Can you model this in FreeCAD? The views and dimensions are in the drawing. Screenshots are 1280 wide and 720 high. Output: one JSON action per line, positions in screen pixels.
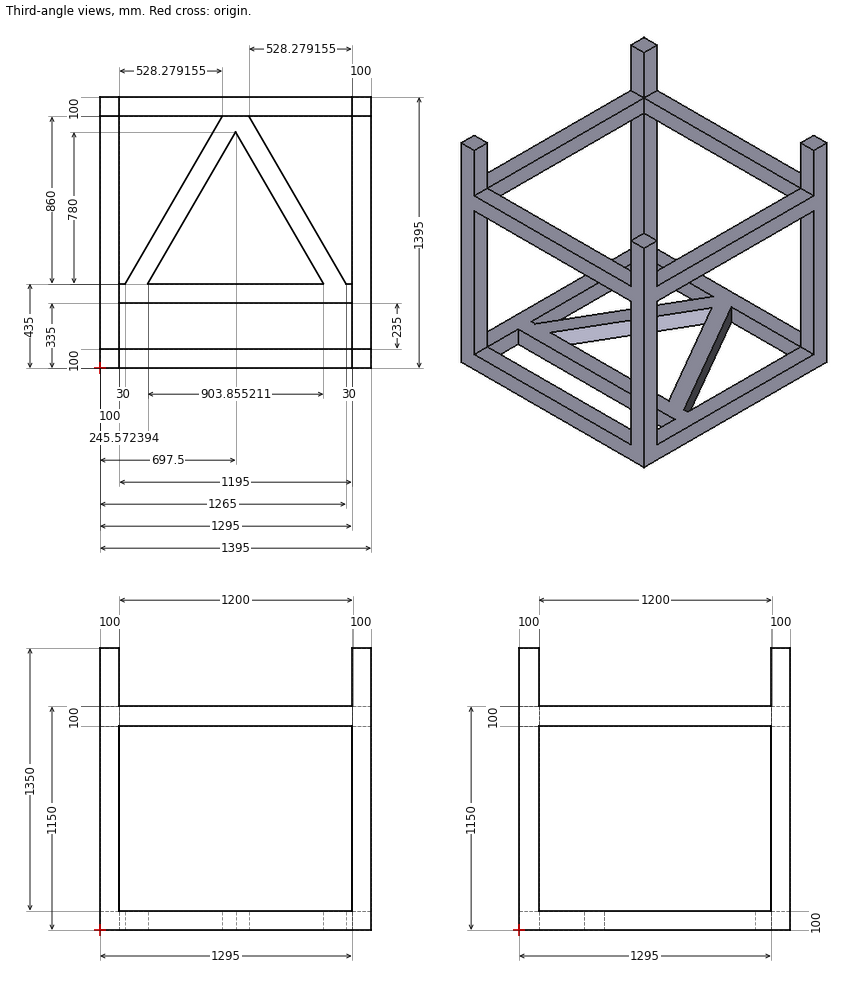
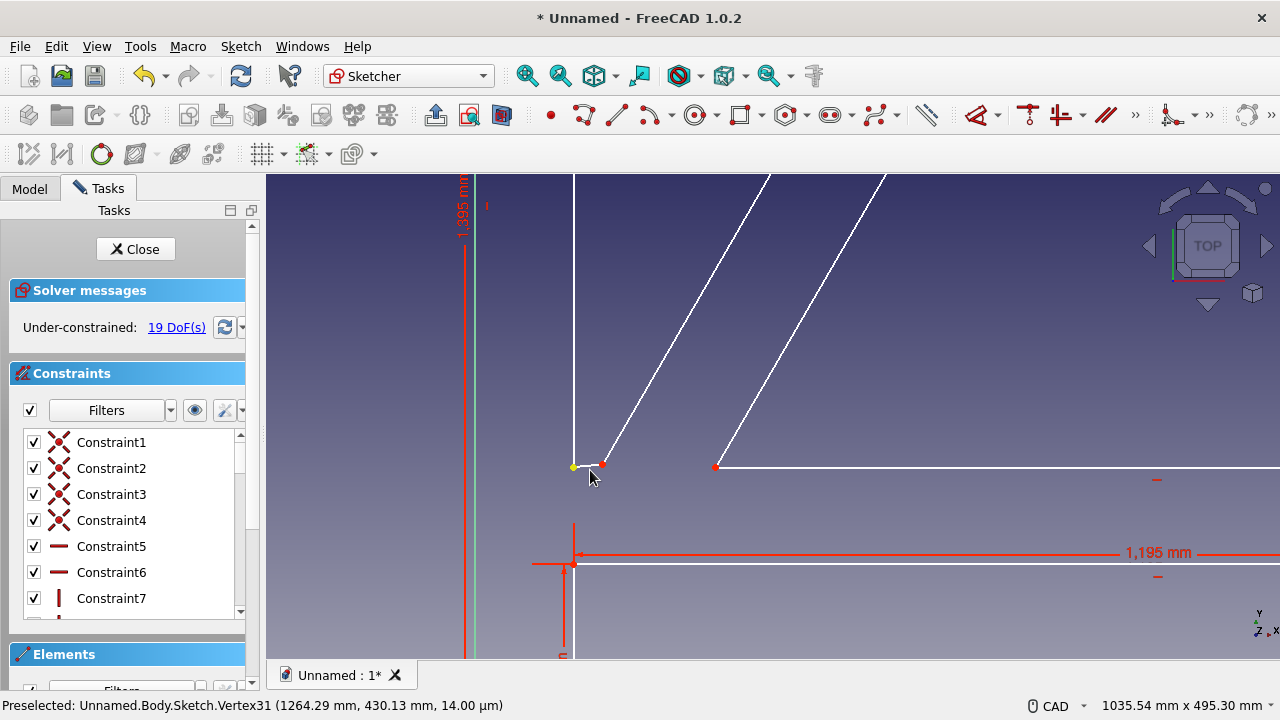
{"action": "left_click", "coordinate": [588, 466]}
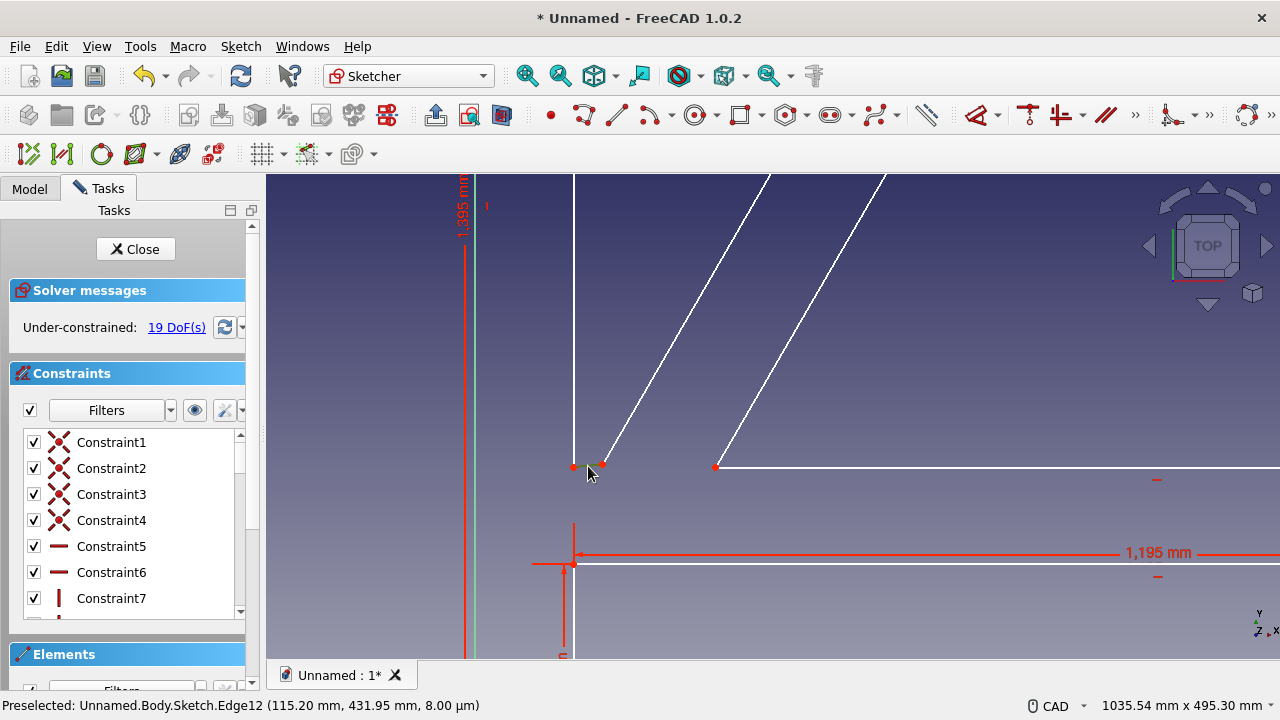
{"action": "left_click", "coordinate": [1082, 116]}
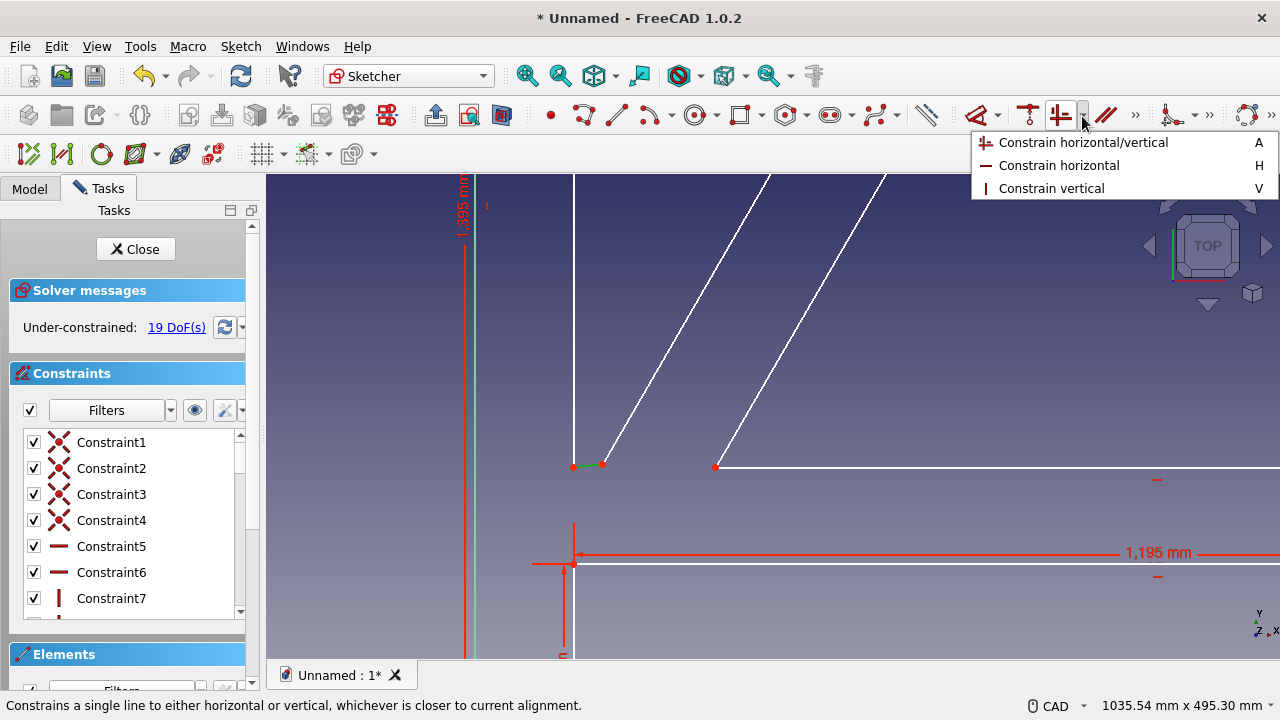
{"action": "left_click", "coordinate": [1125, 166]}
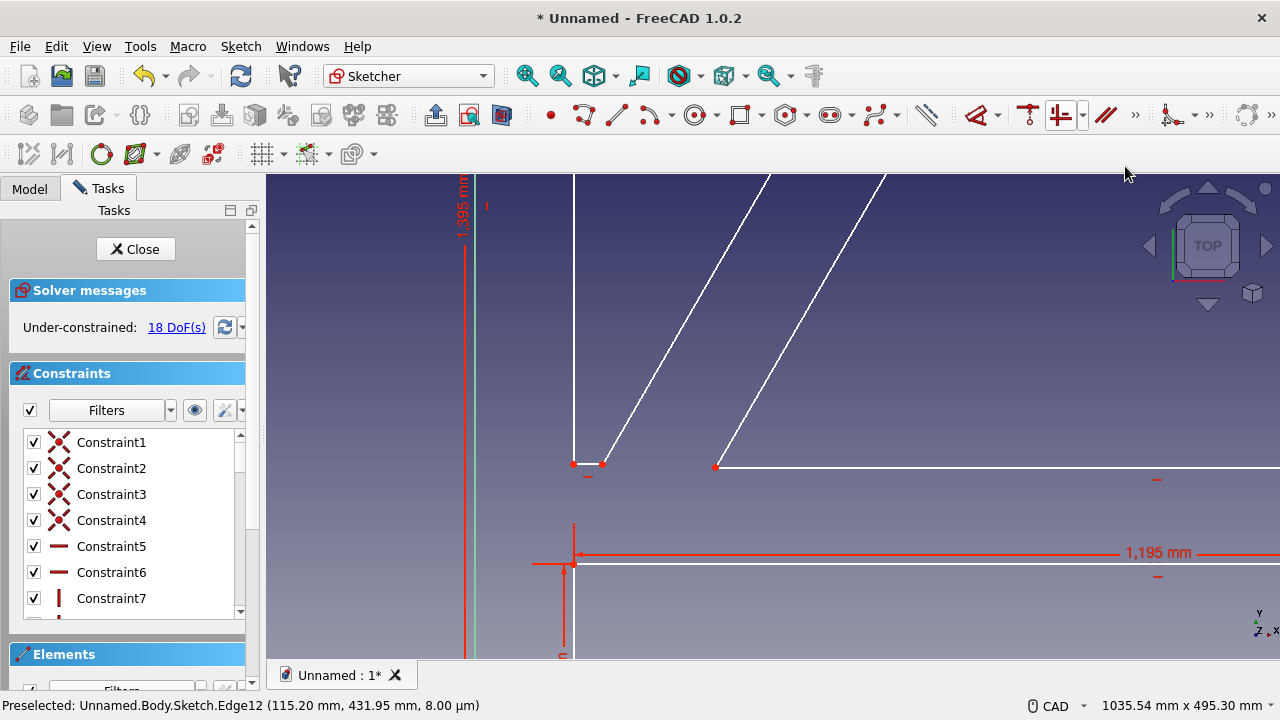
{"action": "scroll", "coordinate": [590, 470], "scroll_direction": "down", "scroll_amount": 8}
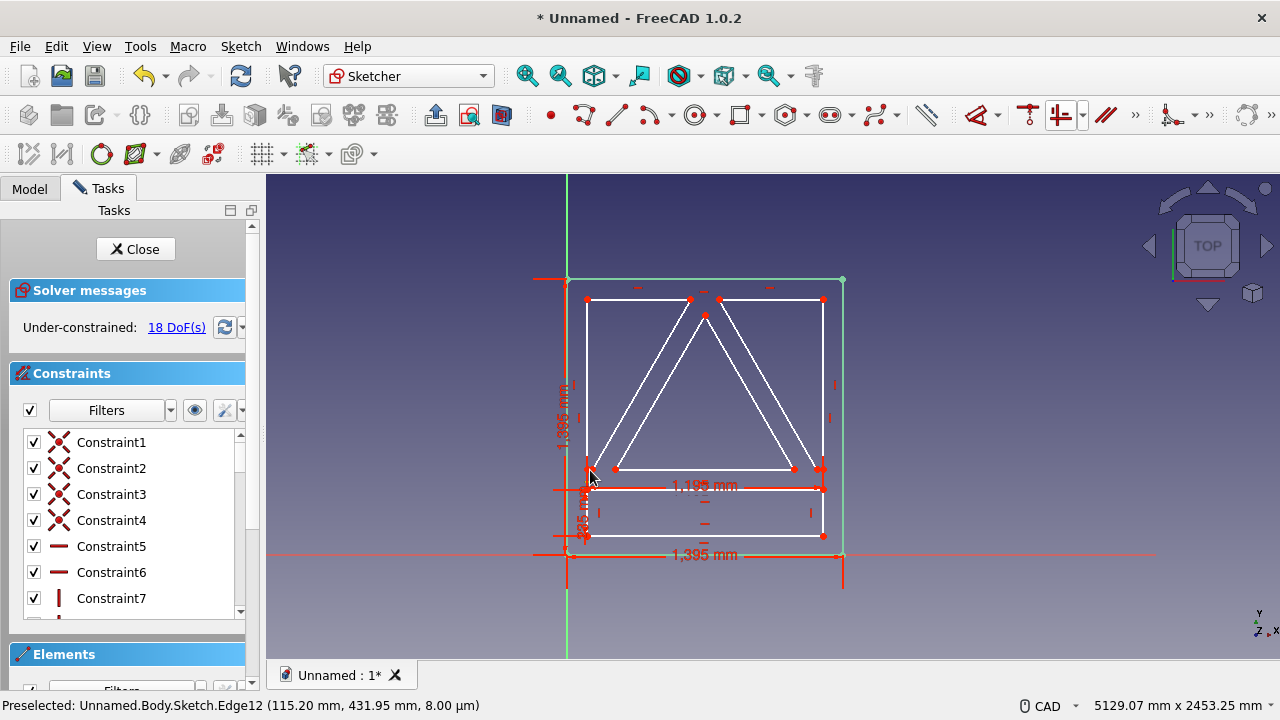
{"action": "scroll", "coordinate": [821, 470], "scroll_direction": "up", "scroll_amount": 9}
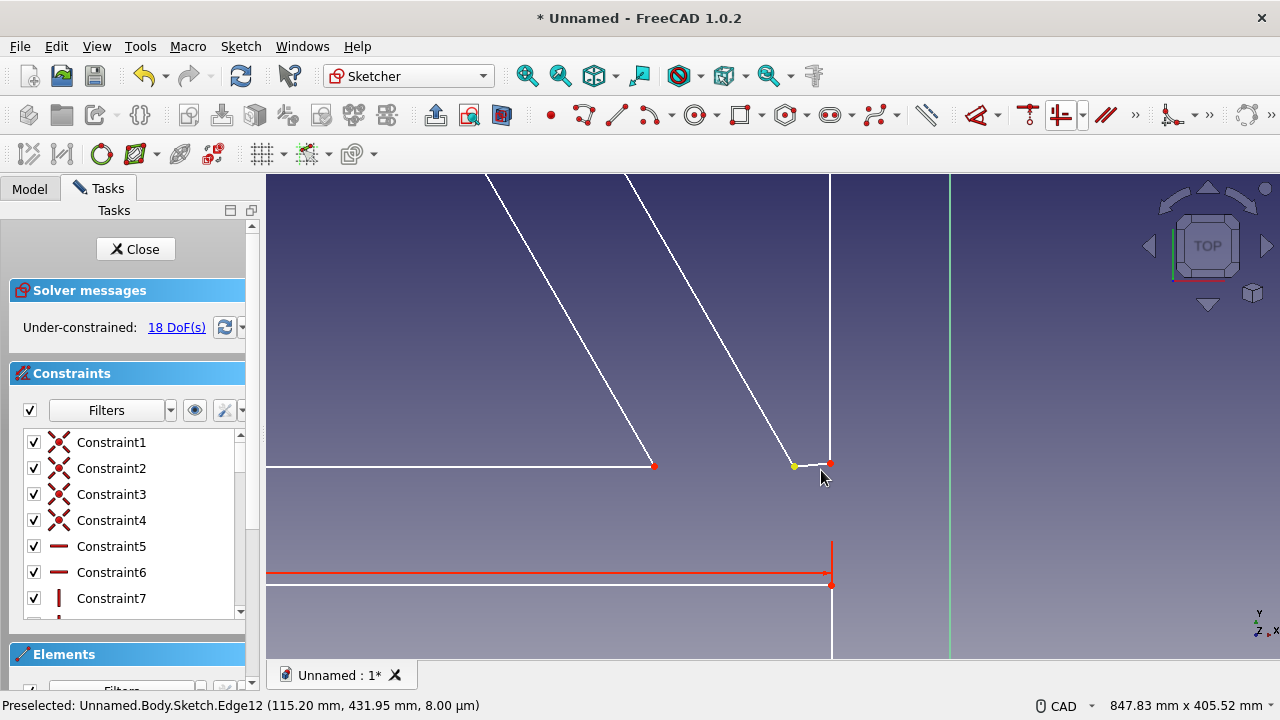
{"action": "left_click", "coordinate": [816, 465]}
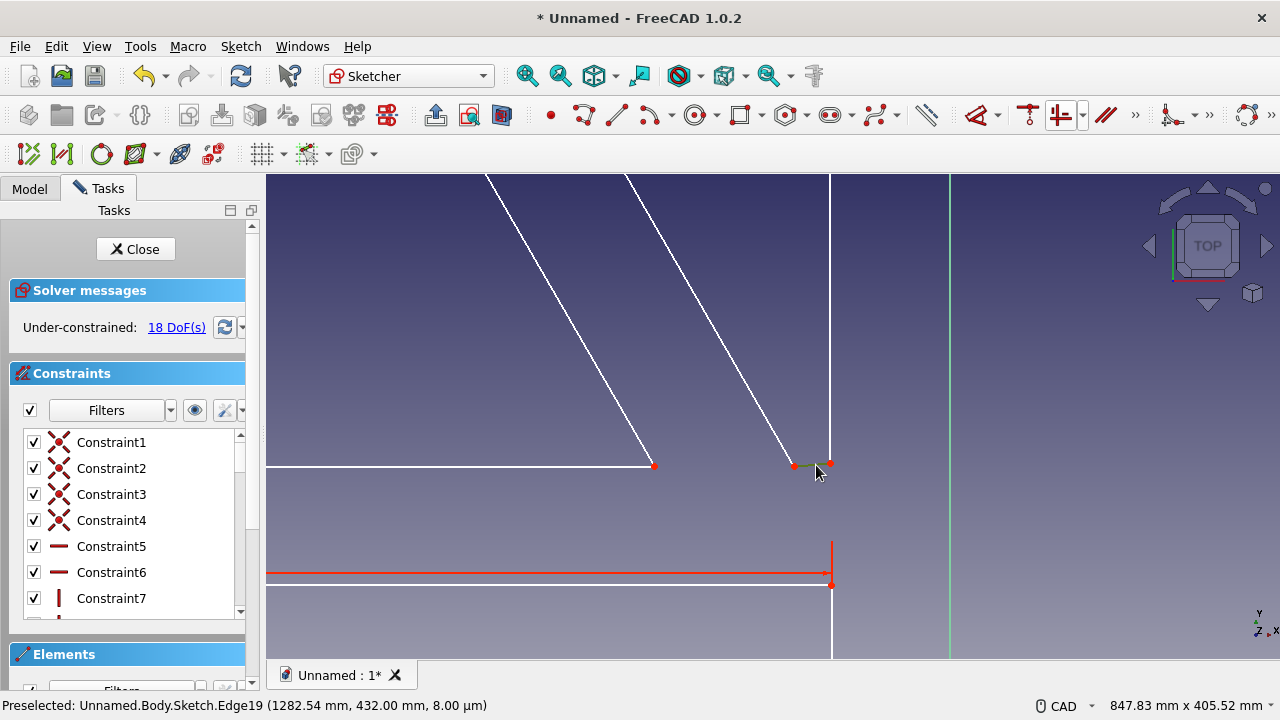
{"action": "left_click", "coordinate": [1082, 116]}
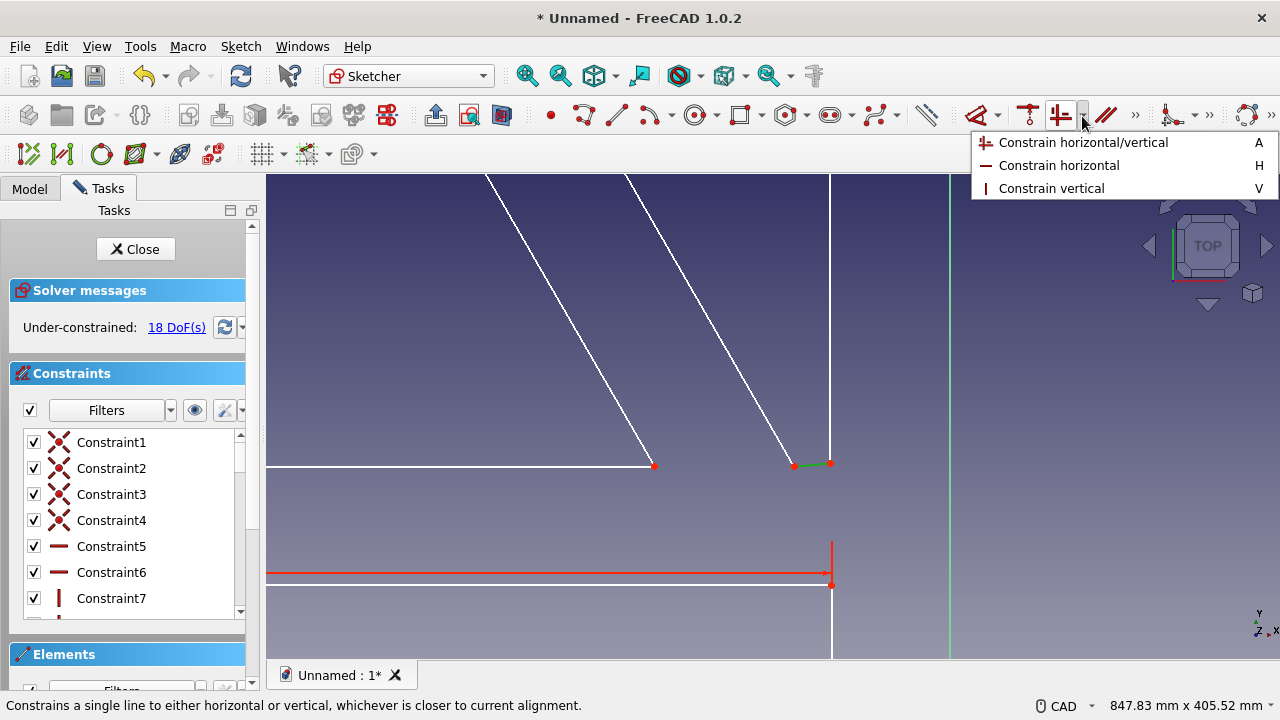
{"action": "left_click", "coordinate": [1125, 166]}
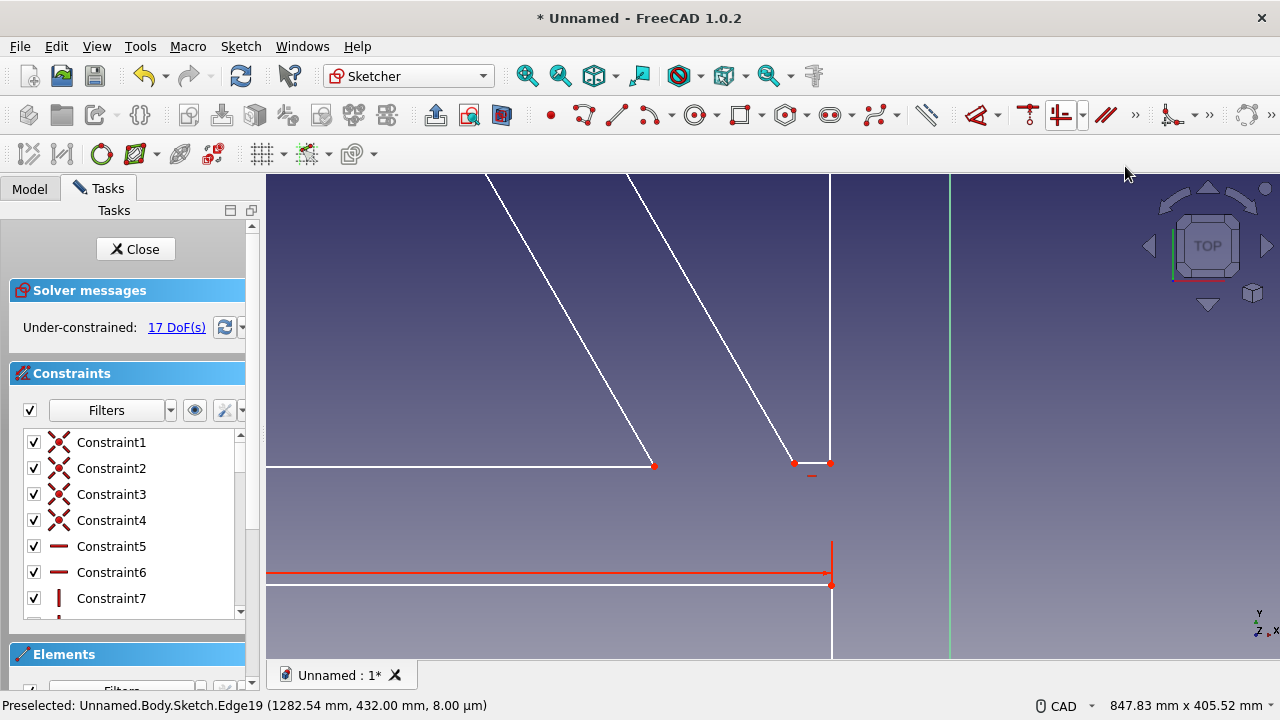
{"action": "scroll", "coordinate": [821, 470], "scroll_direction": "down", "scroll_amount": 9}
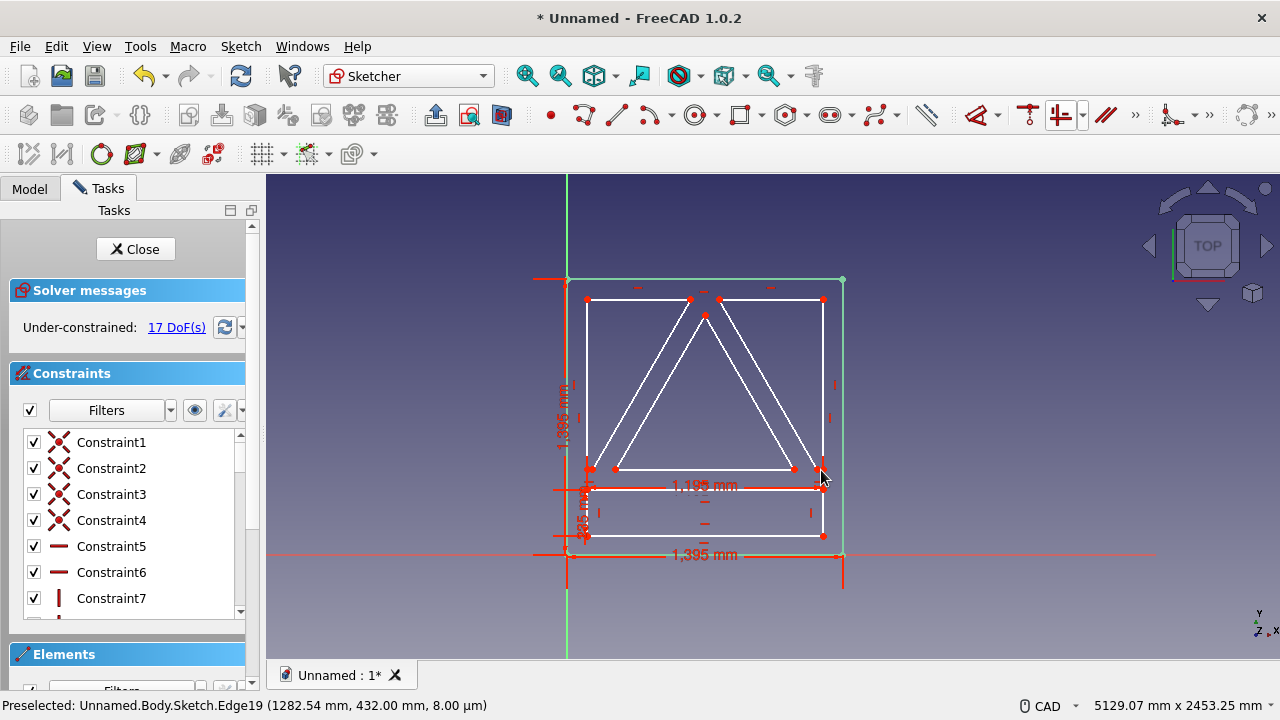
{"action": "scroll", "coordinate": [591, 469], "scroll_direction": "up", "scroll_amount": 11}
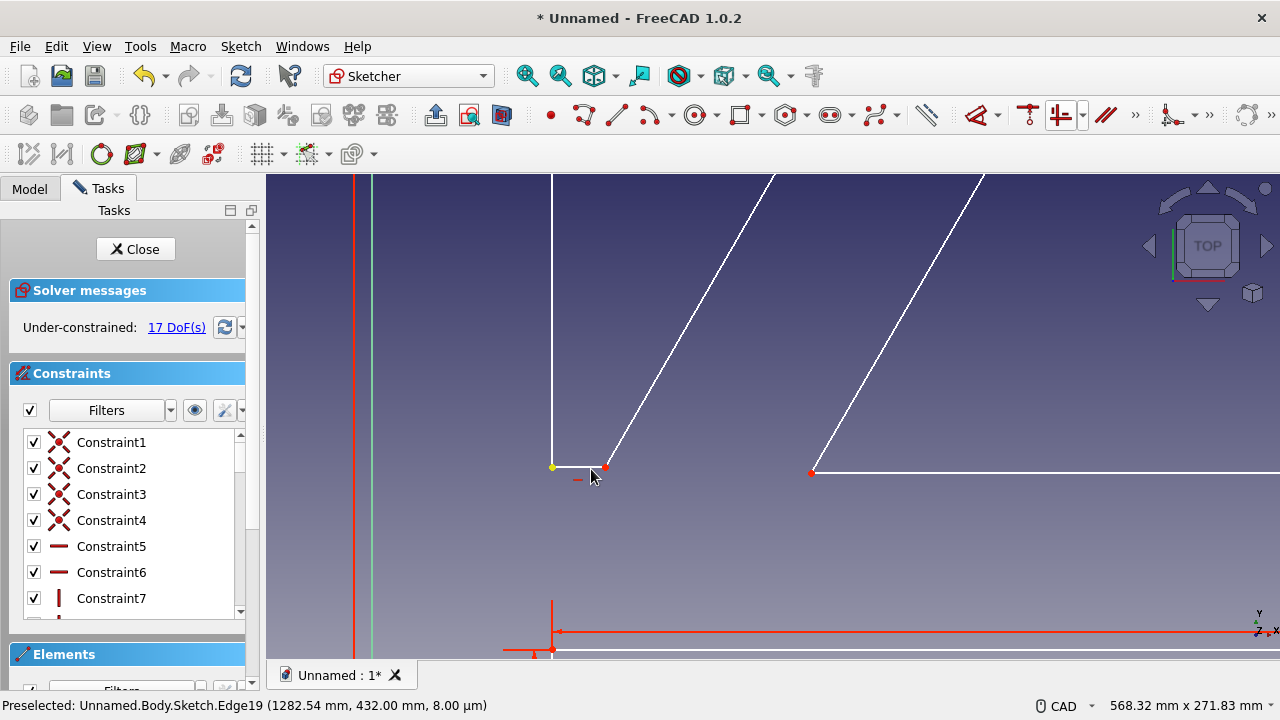
{"action": "left_click", "coordinate": [589, 467]}